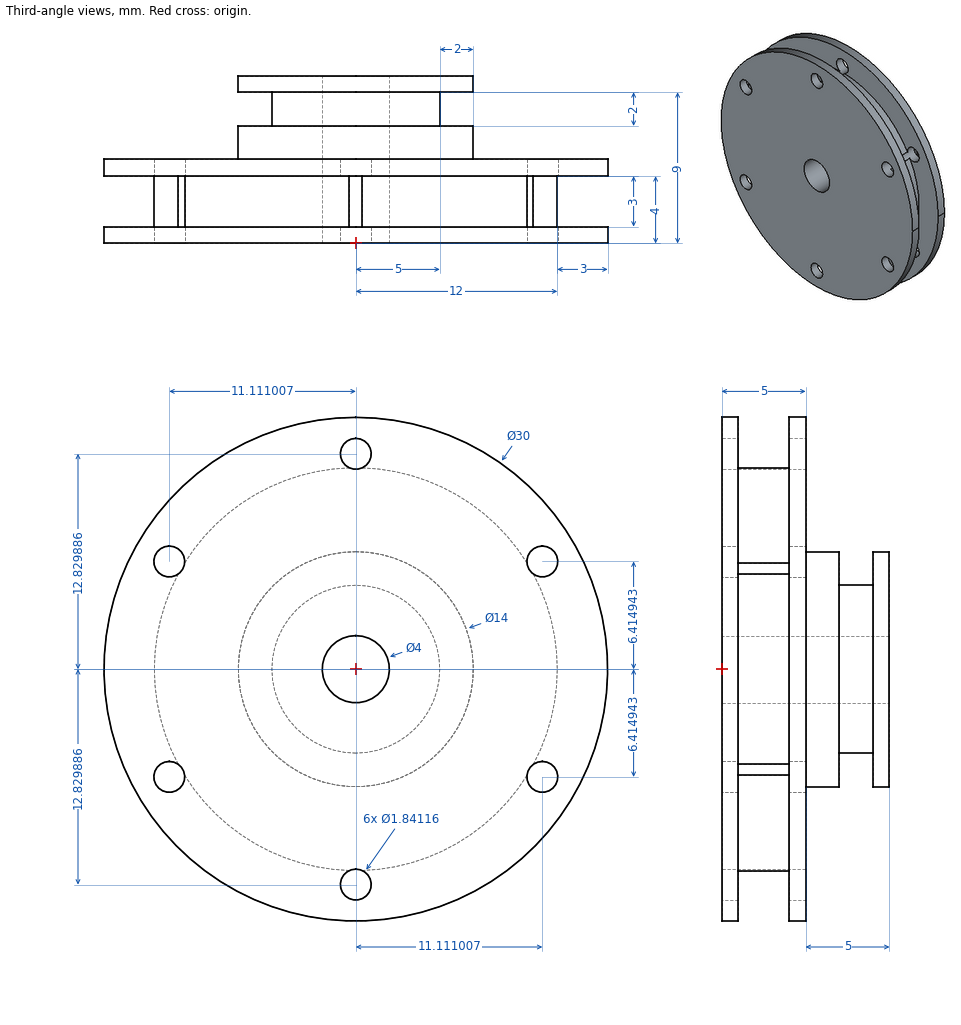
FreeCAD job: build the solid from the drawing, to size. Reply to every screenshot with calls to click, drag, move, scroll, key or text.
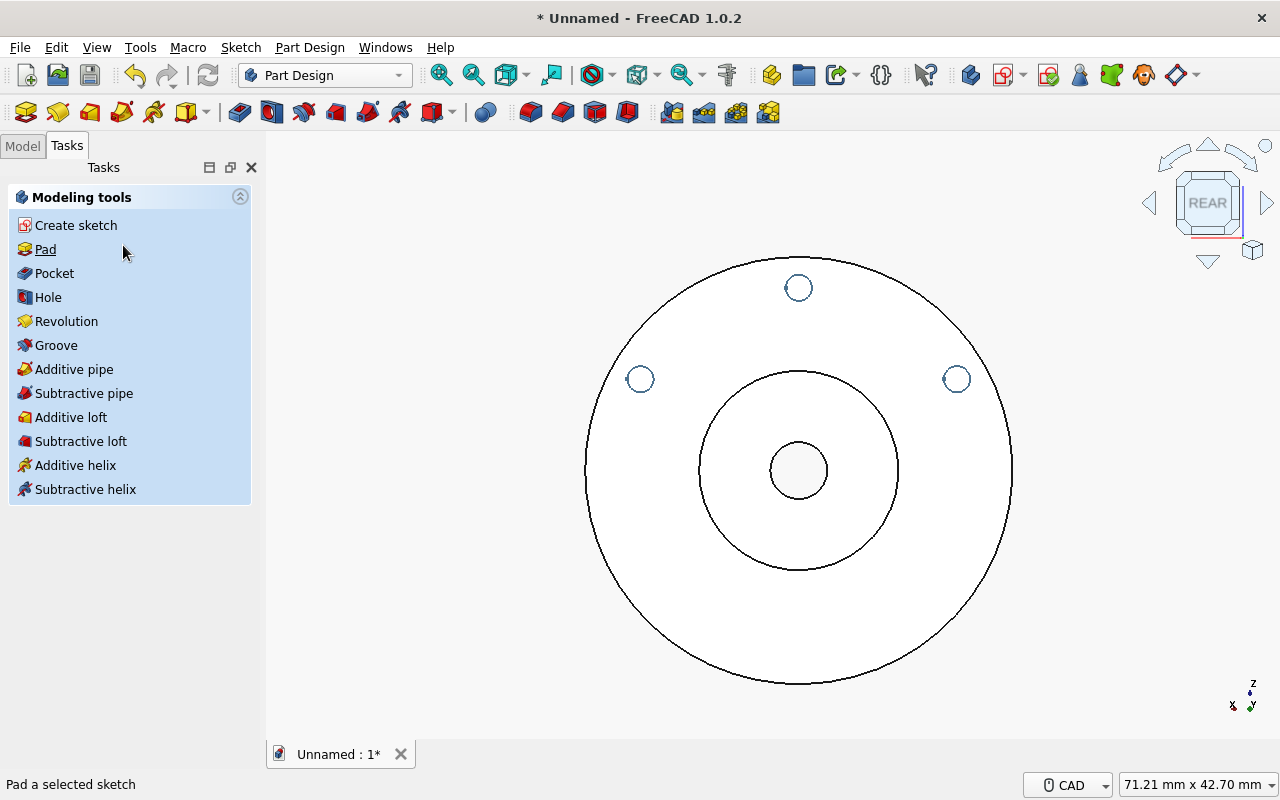
click(240, 112)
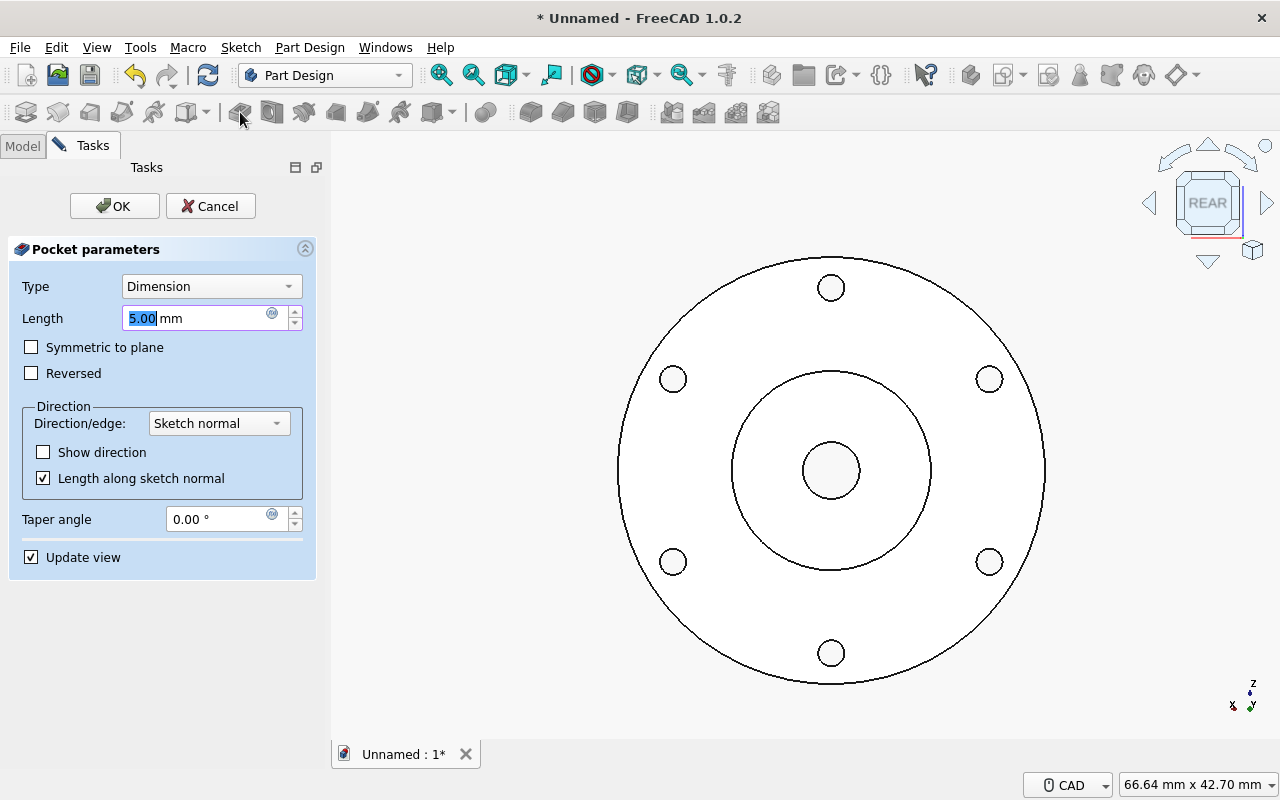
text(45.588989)
key(Tab)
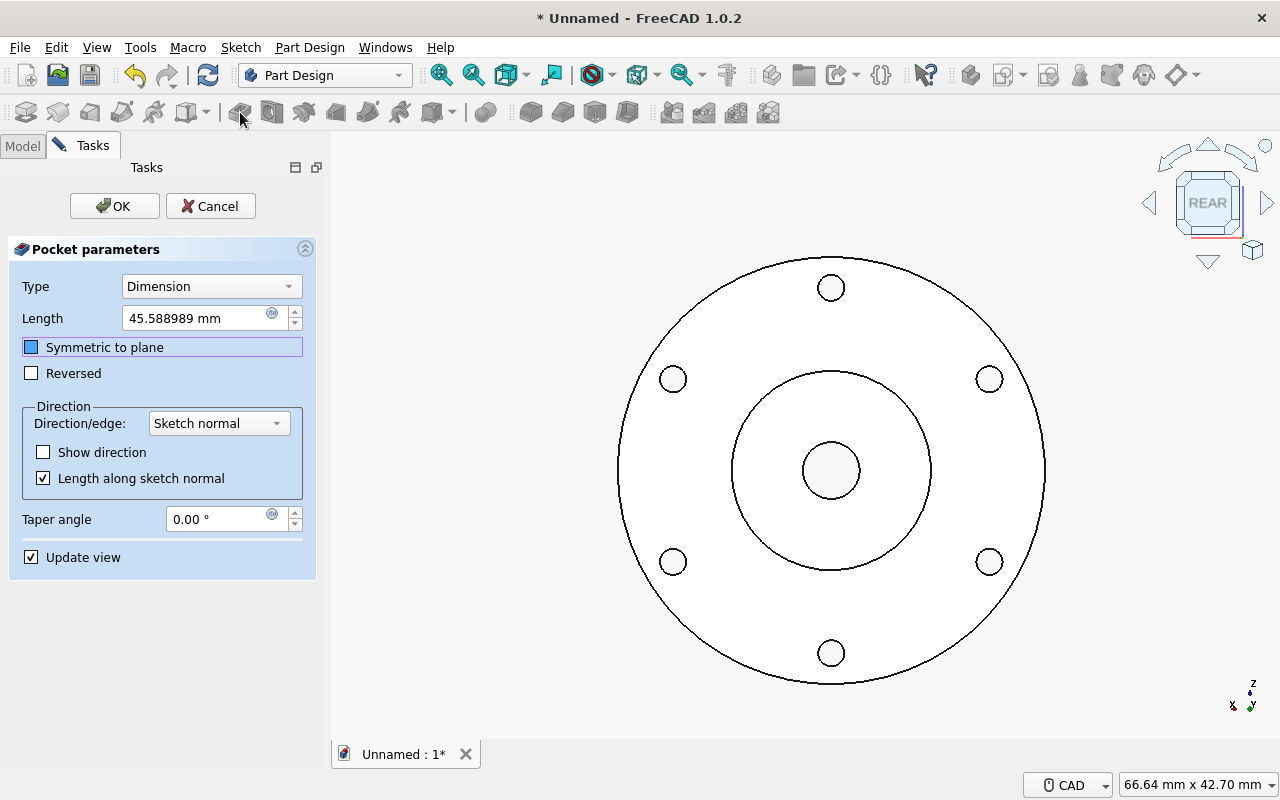
click(30, 347)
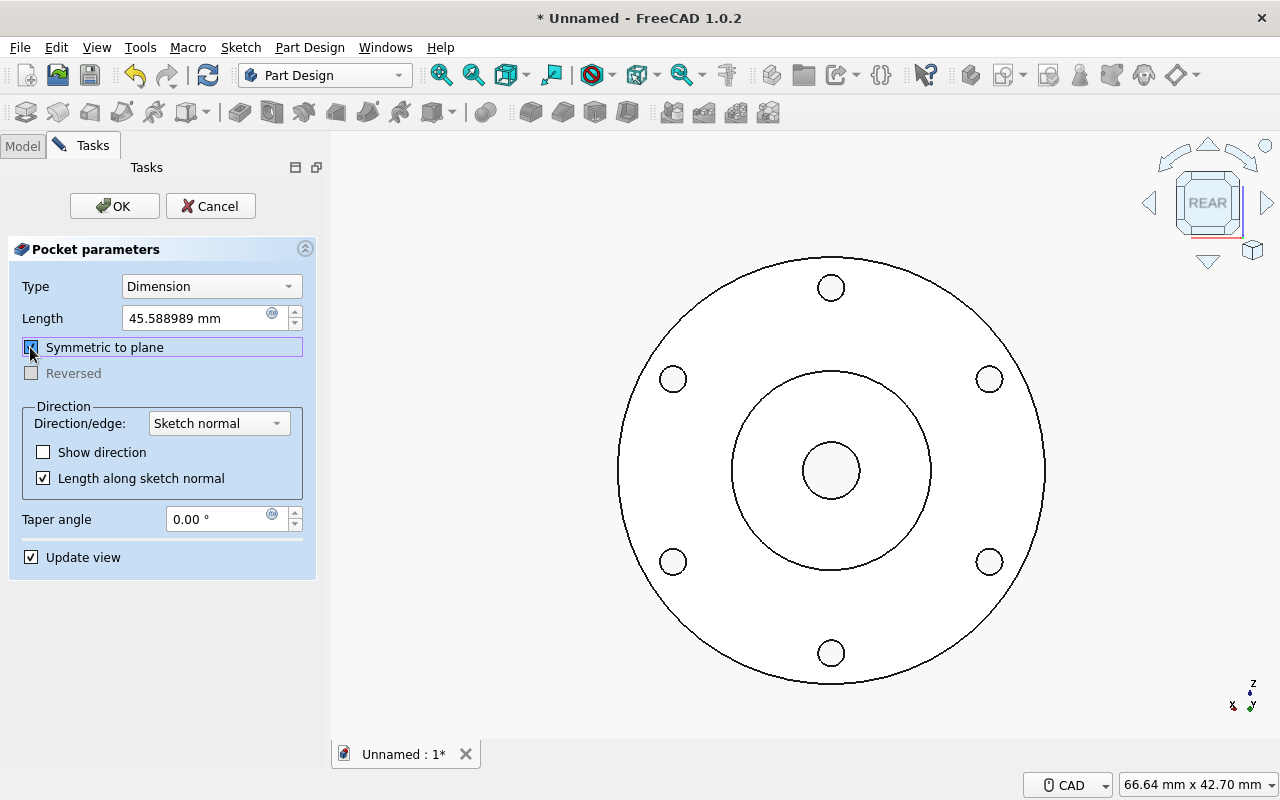
click(115, 206)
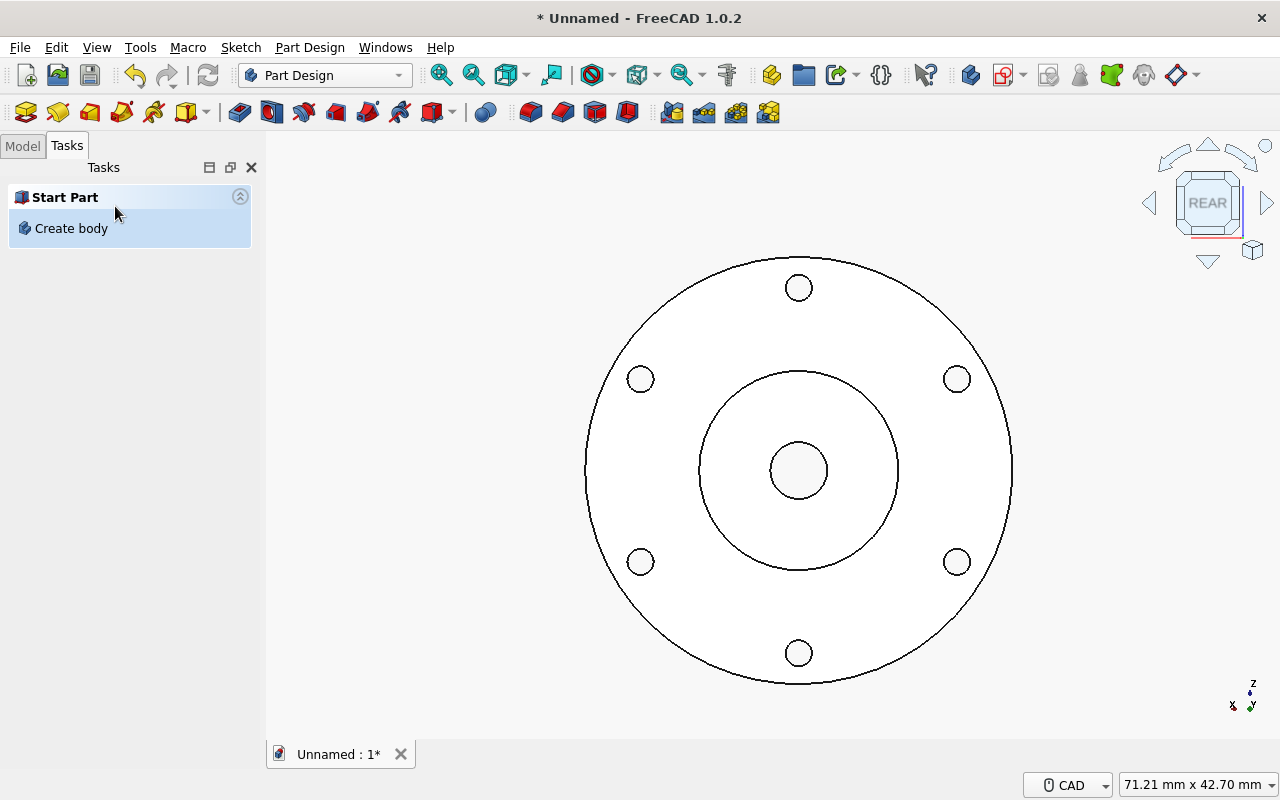
key(0)